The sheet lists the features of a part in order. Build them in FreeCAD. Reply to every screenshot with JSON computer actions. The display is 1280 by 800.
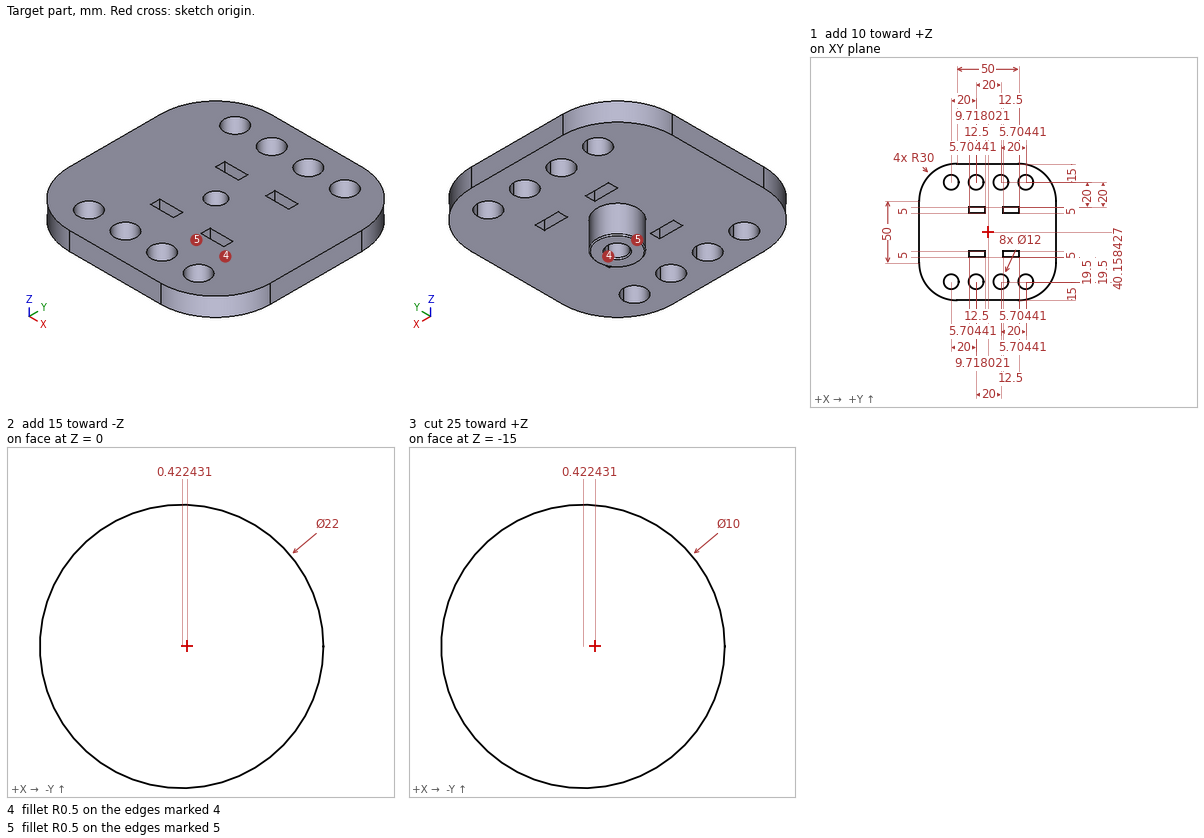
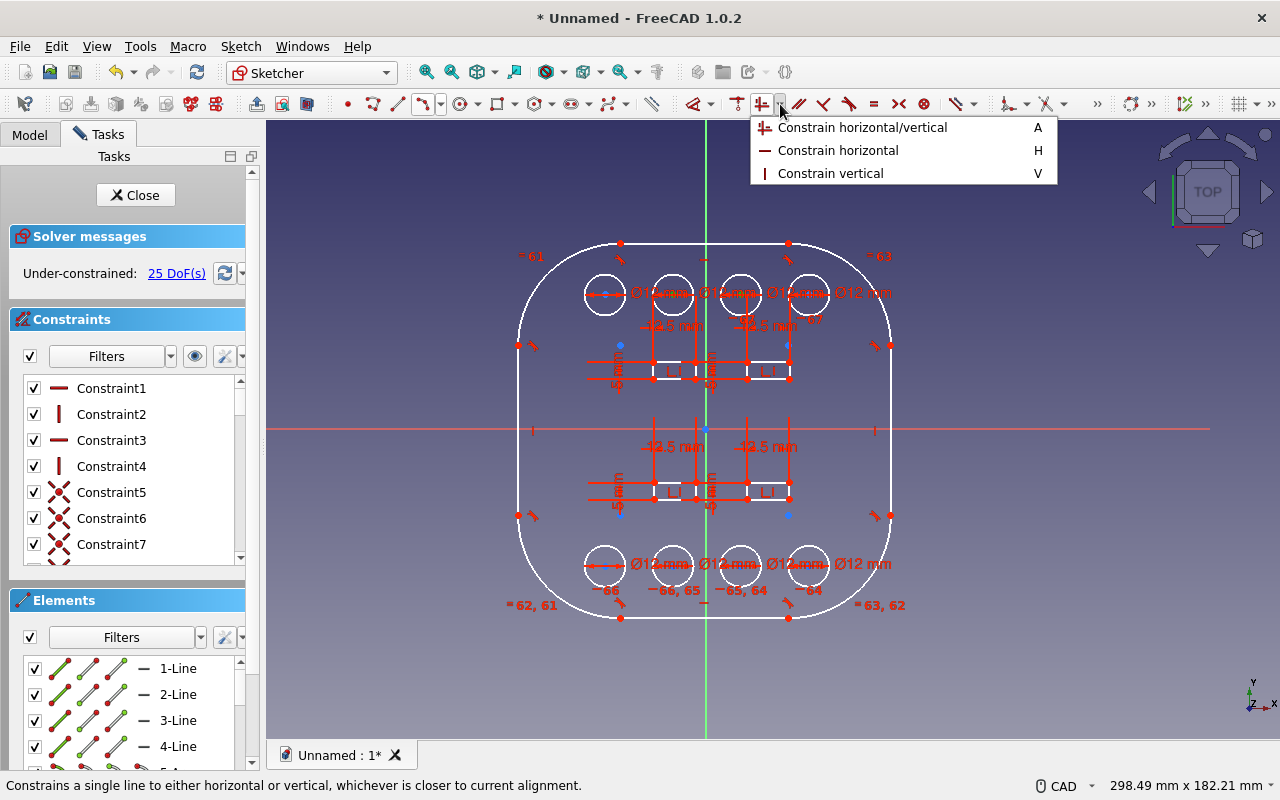
{"action": "left_click", "coordinate": [904, 150]}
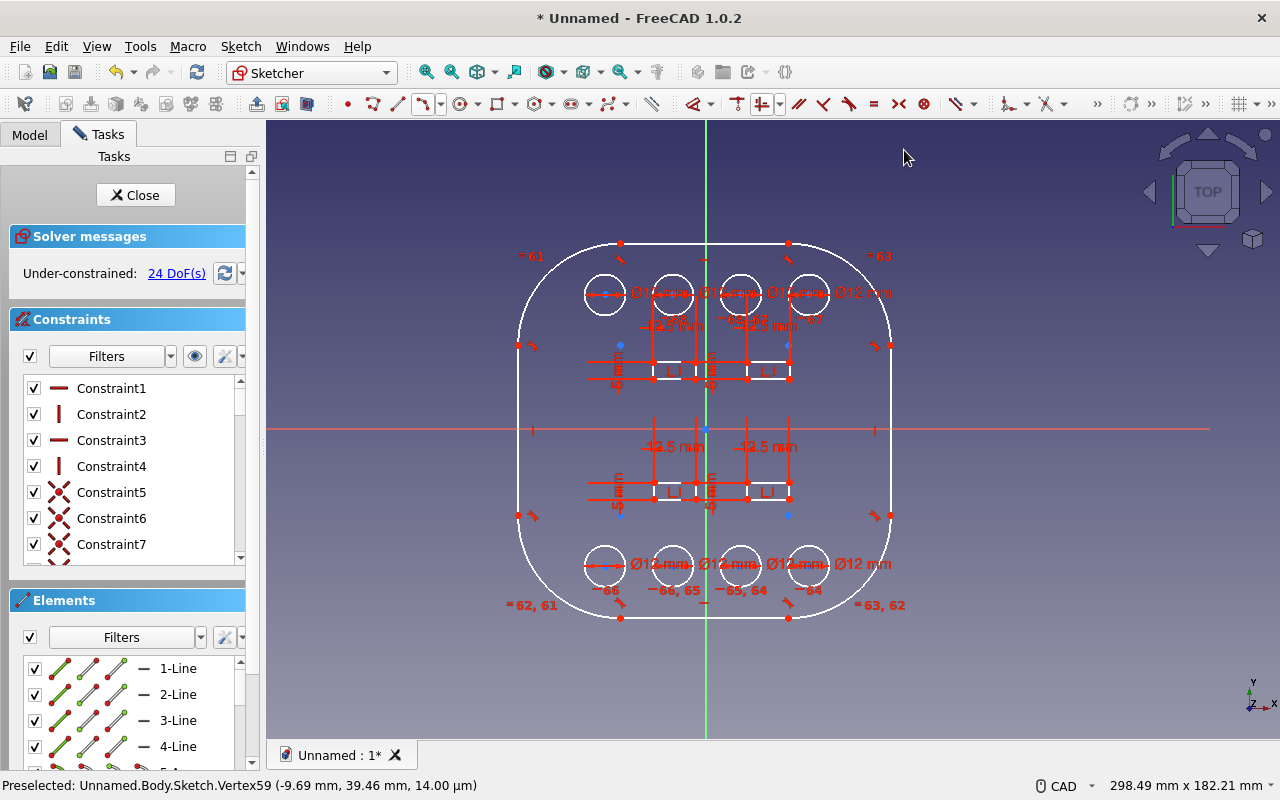
{"action": "left_click", "coordinate": [673, 295]}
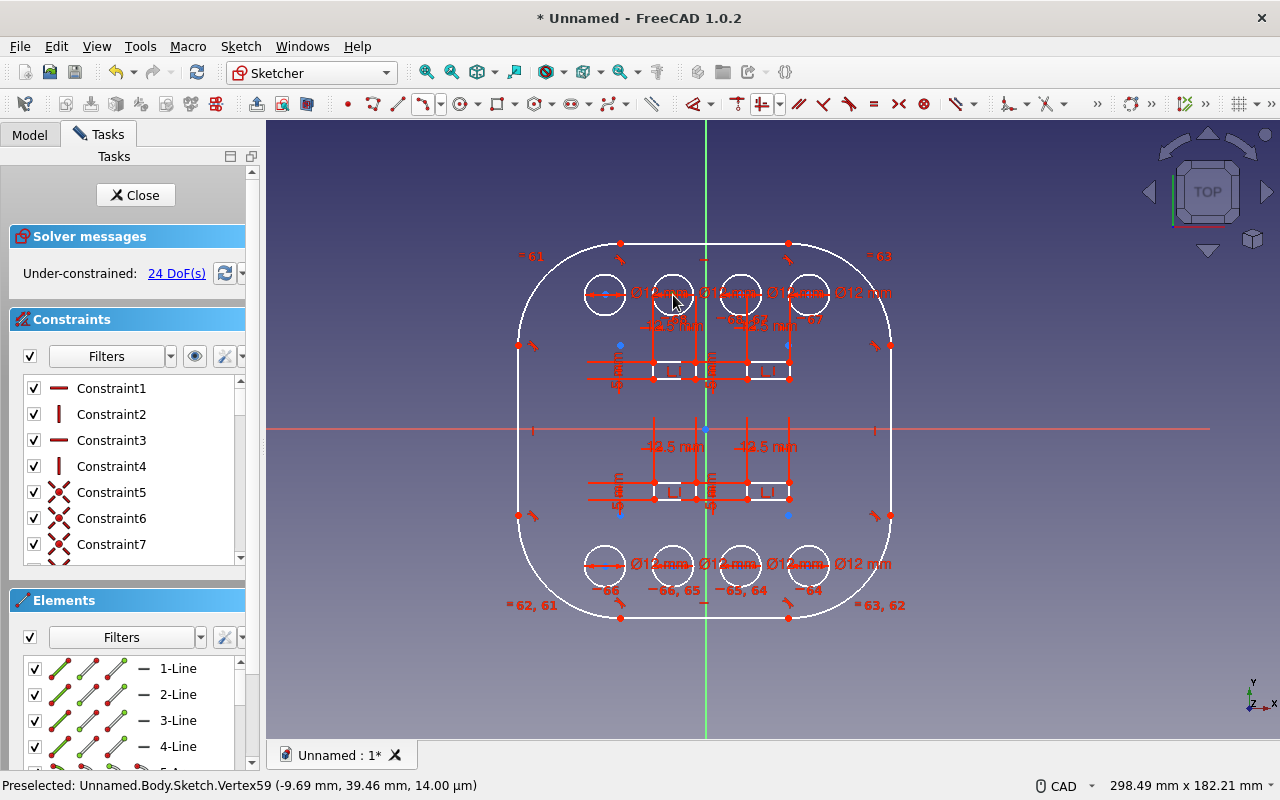
{"action": "left_click", "coordinate": [605, 295]}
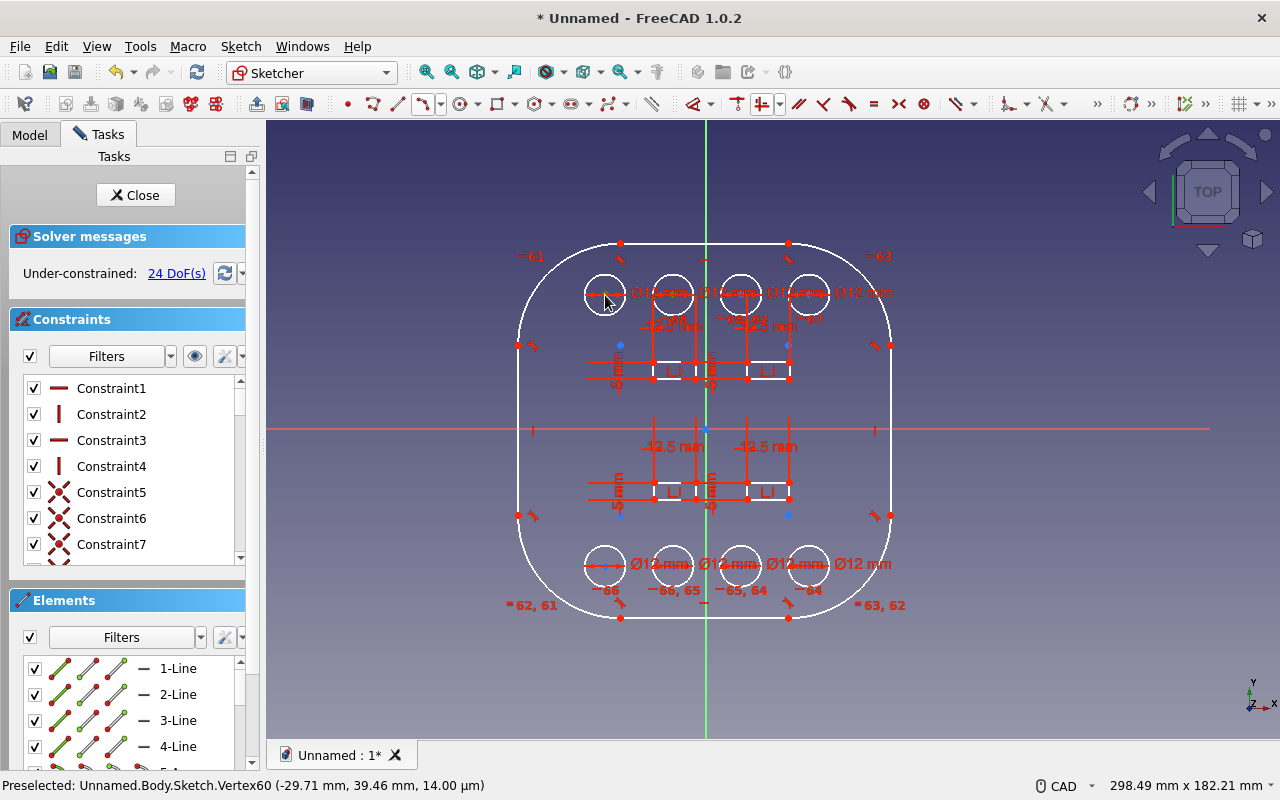
{"action": "key", "text": "h"}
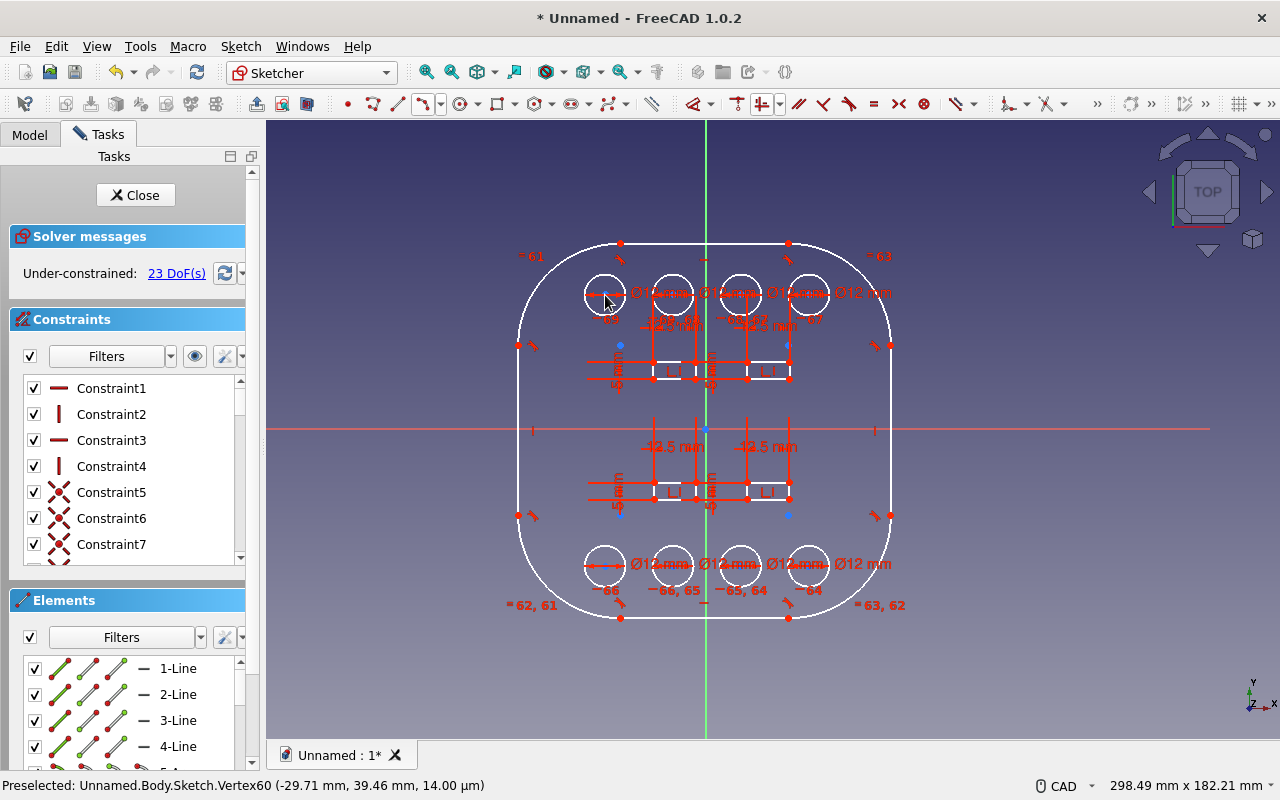
{"action": "left_click", "coordinate": [574, 255]}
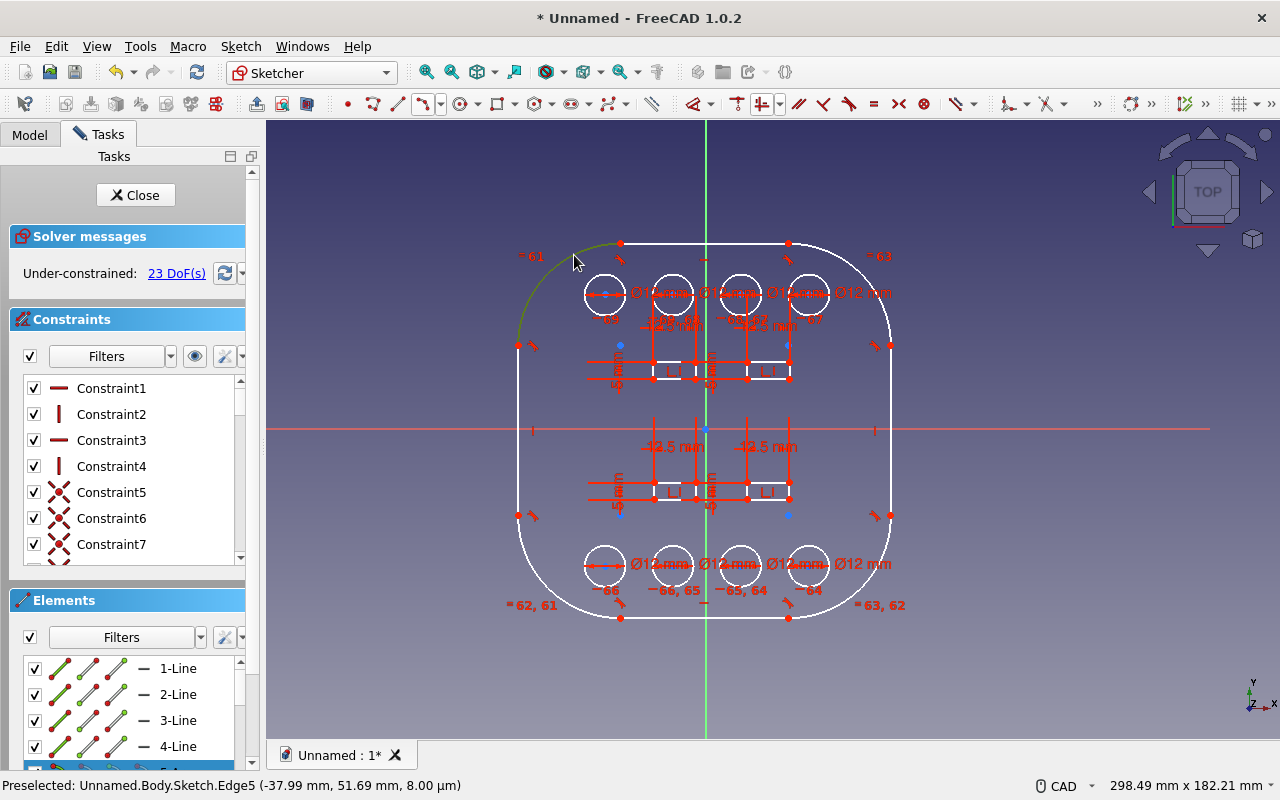
{"action": "left_click", "coordinate": [710, 104]}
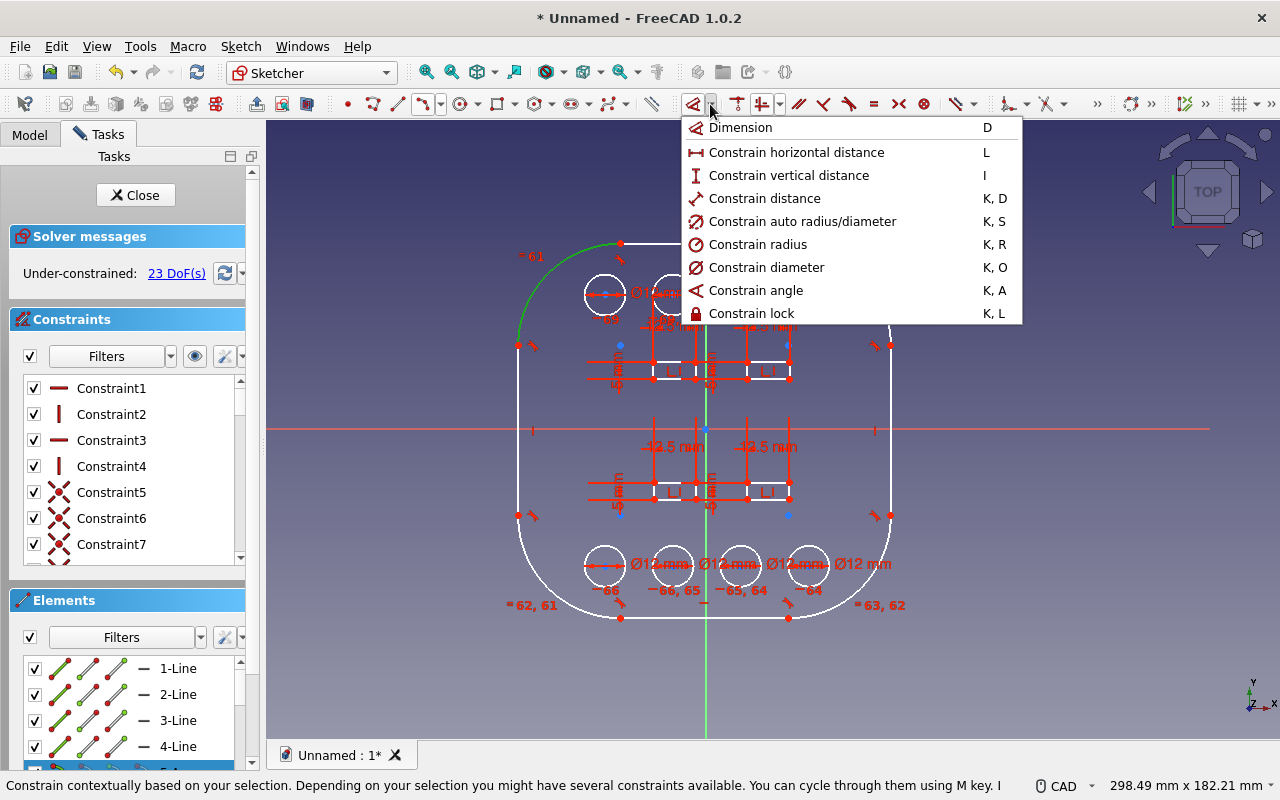
{"action": "left_click", "coordinate": [852, 244]}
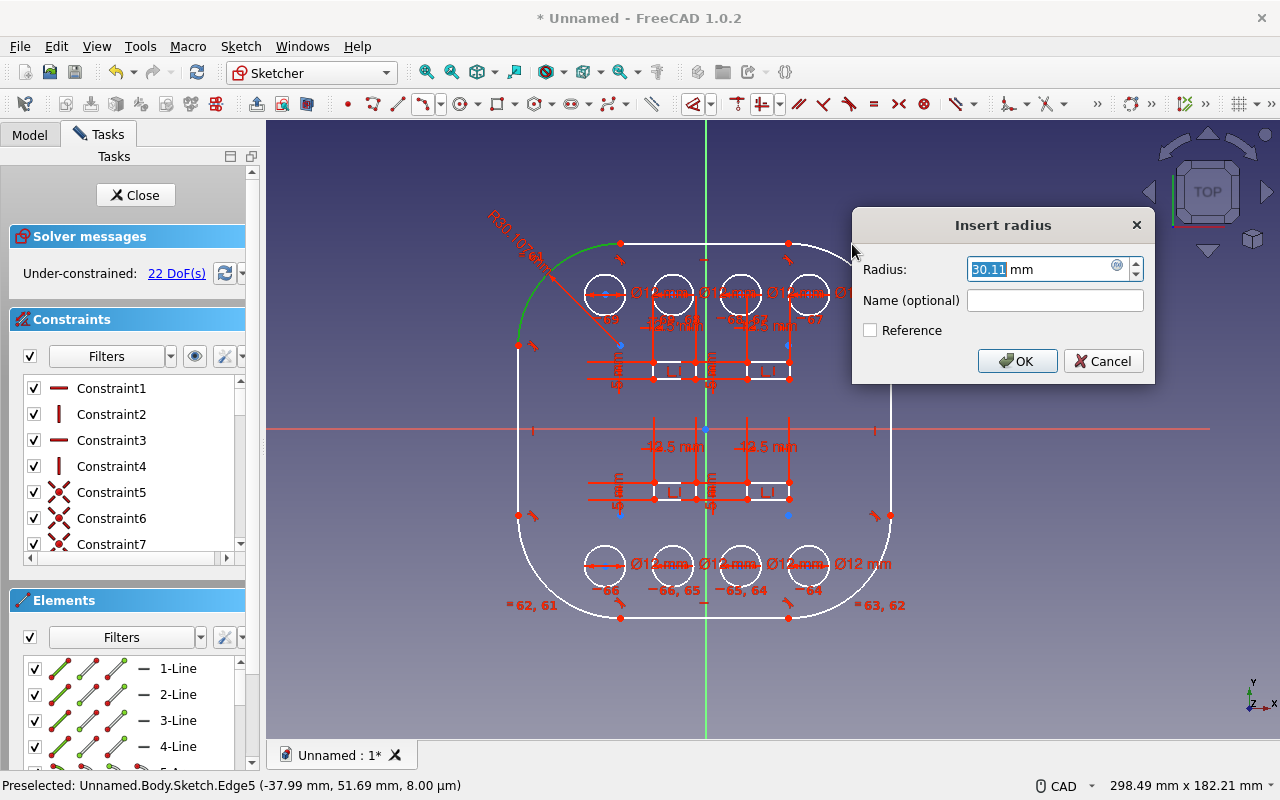
{"action": "type", "text": "30"}
{"action": "key", "text": "Return"}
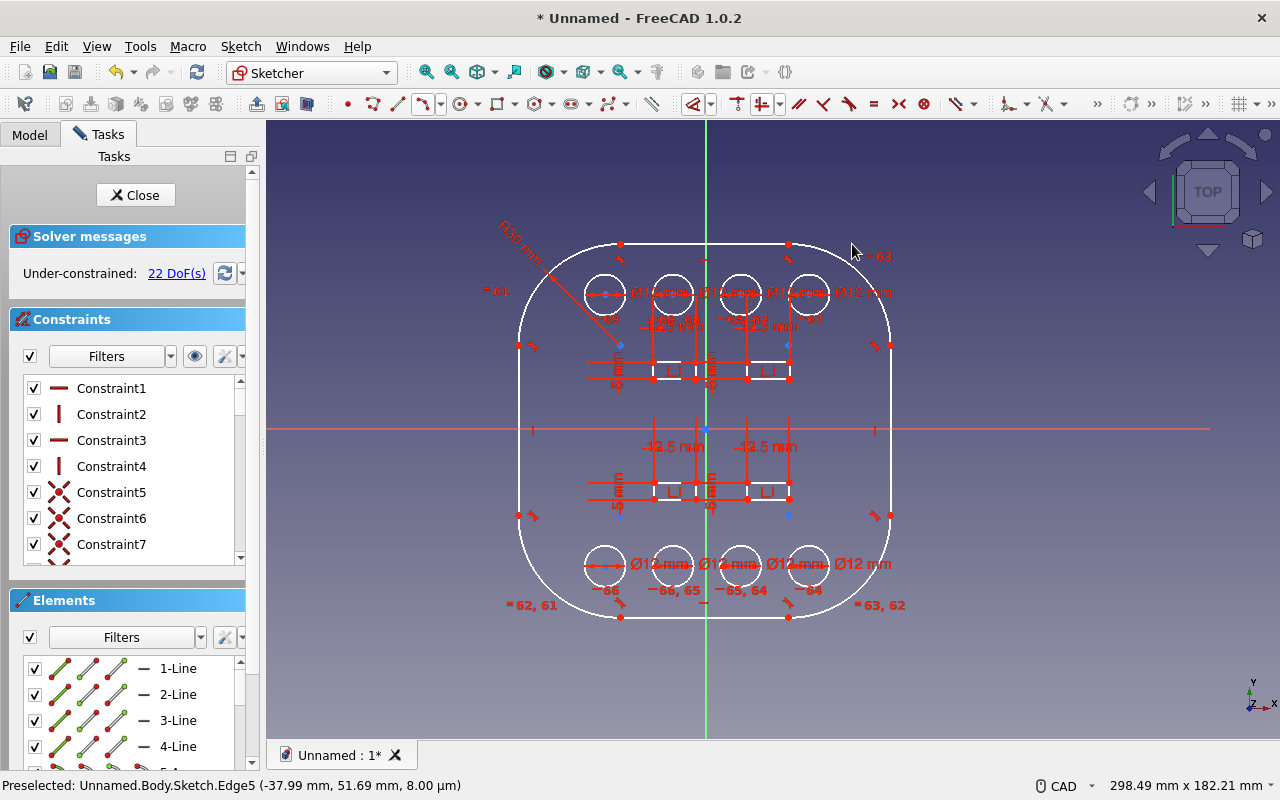
{"action": "left_click", "coordinate": [738, 244]}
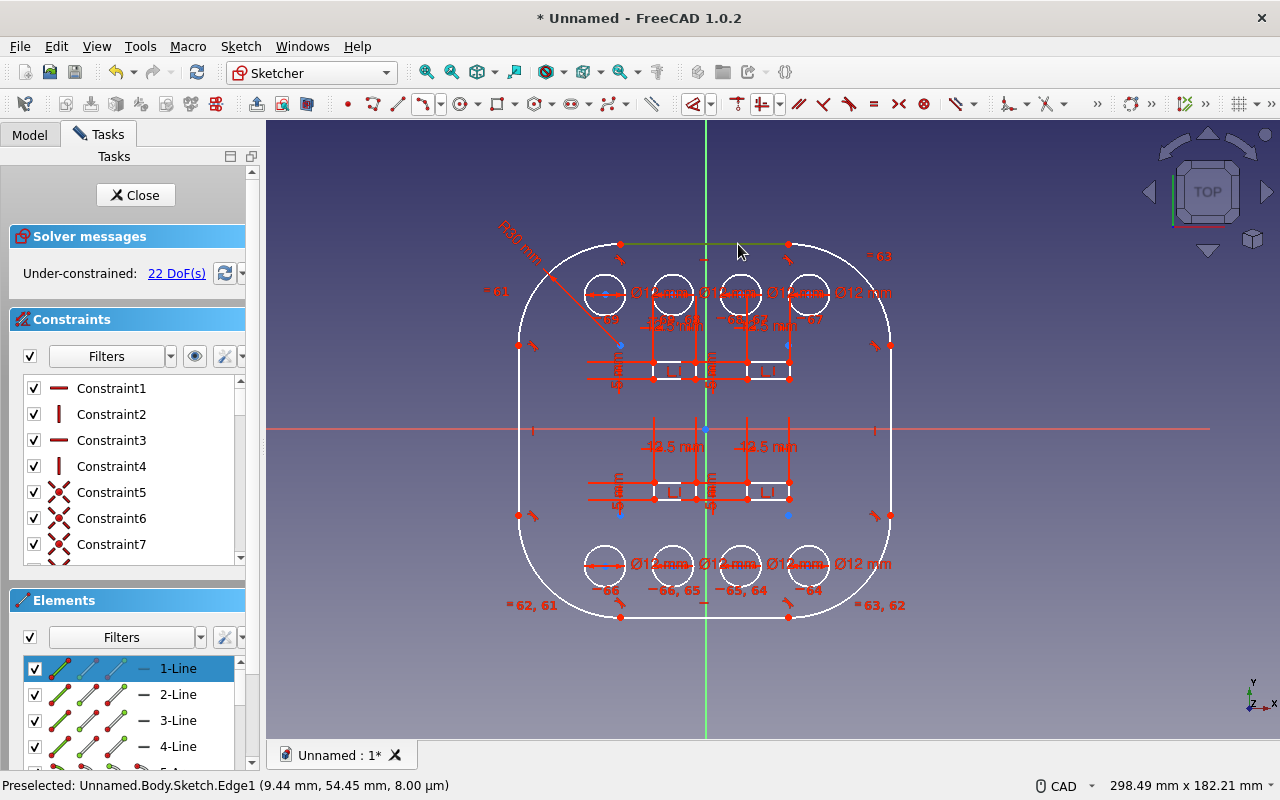
{"action": "key", "text": "l"}